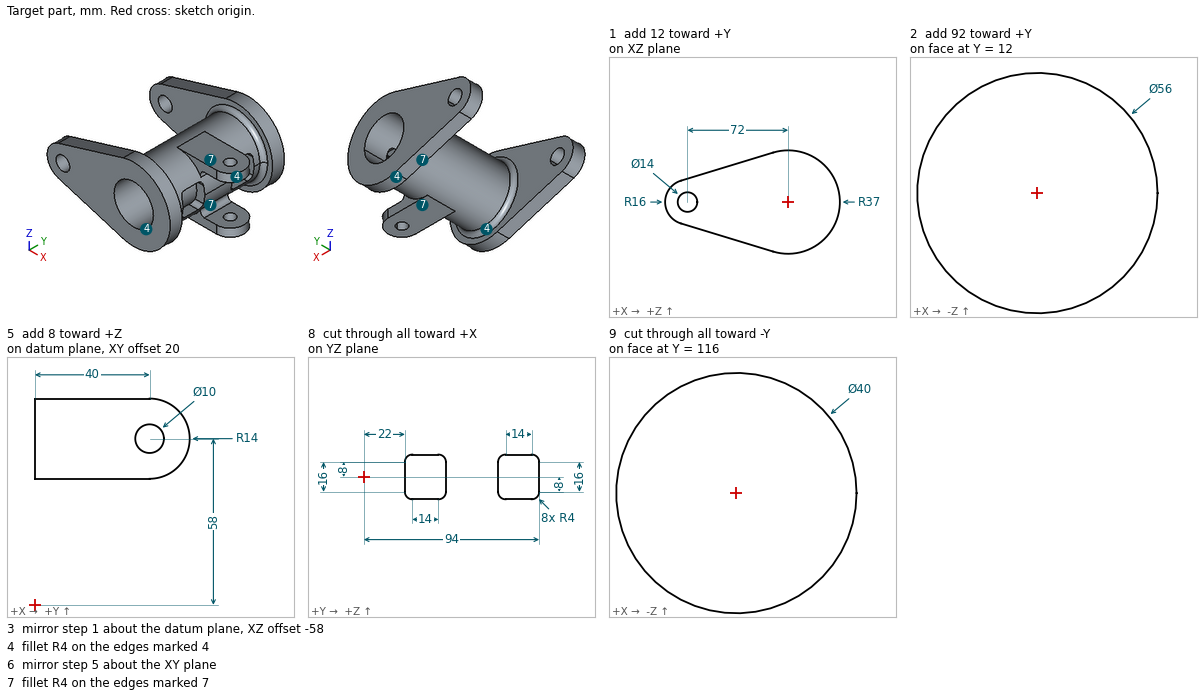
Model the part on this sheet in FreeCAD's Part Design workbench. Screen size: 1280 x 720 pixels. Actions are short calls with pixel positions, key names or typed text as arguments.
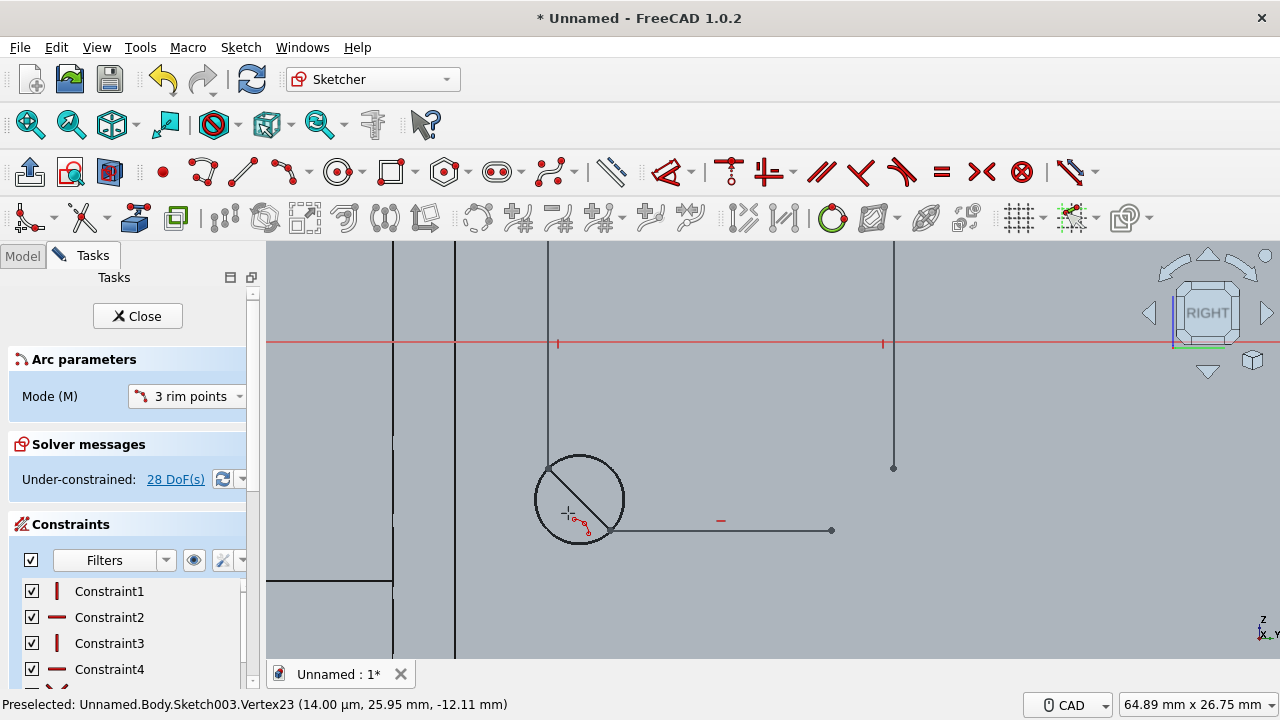
click(568, 511)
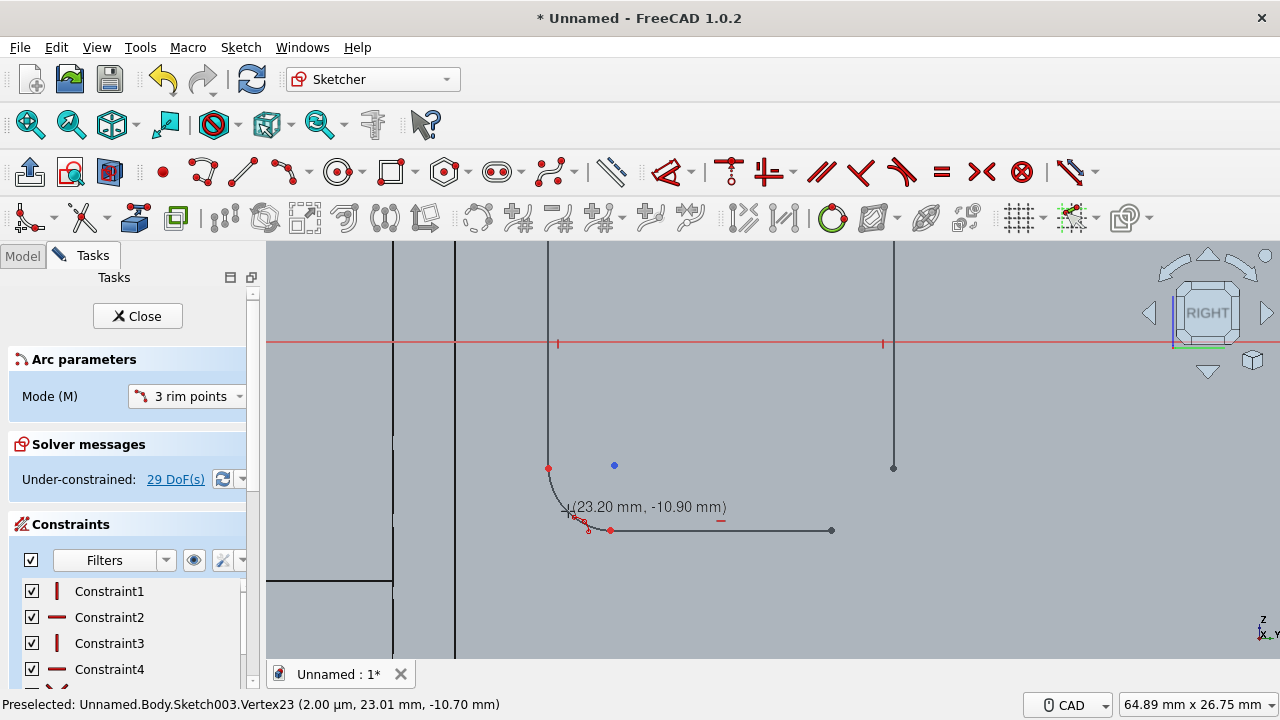
click(831, 531)
click(894, 468)
click(875, 511)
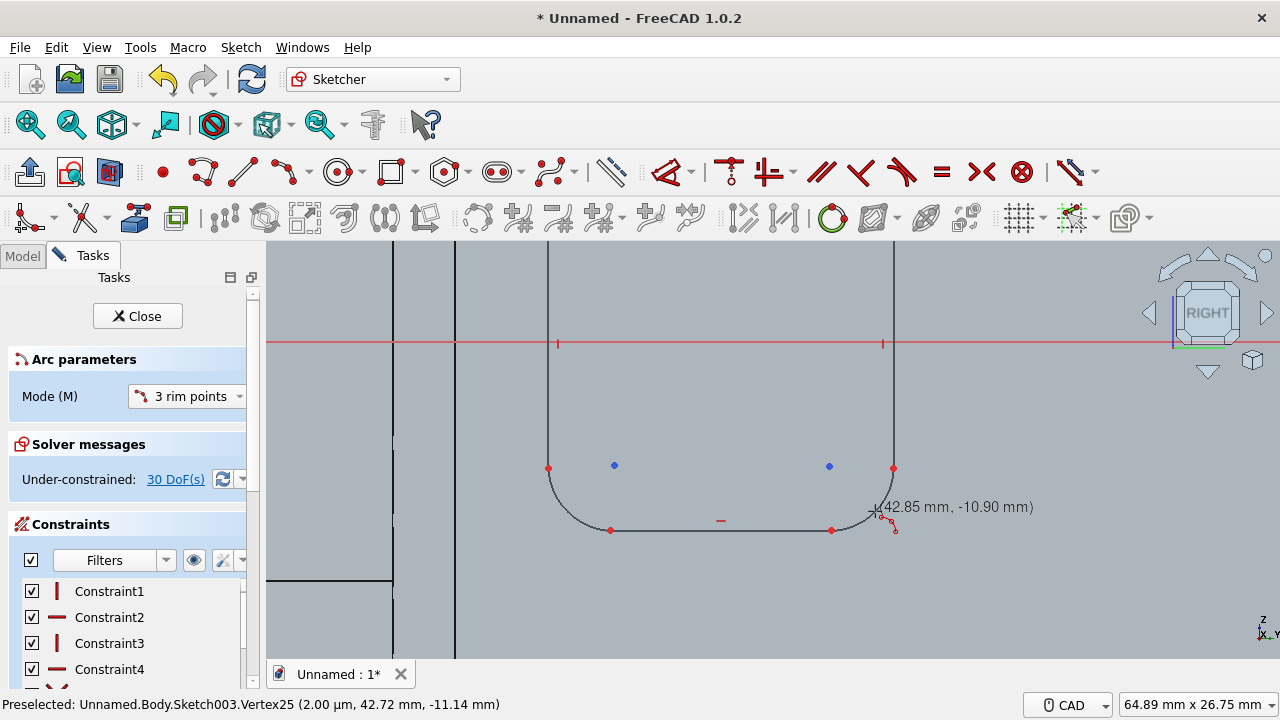
scroll(567, 513, down, 5)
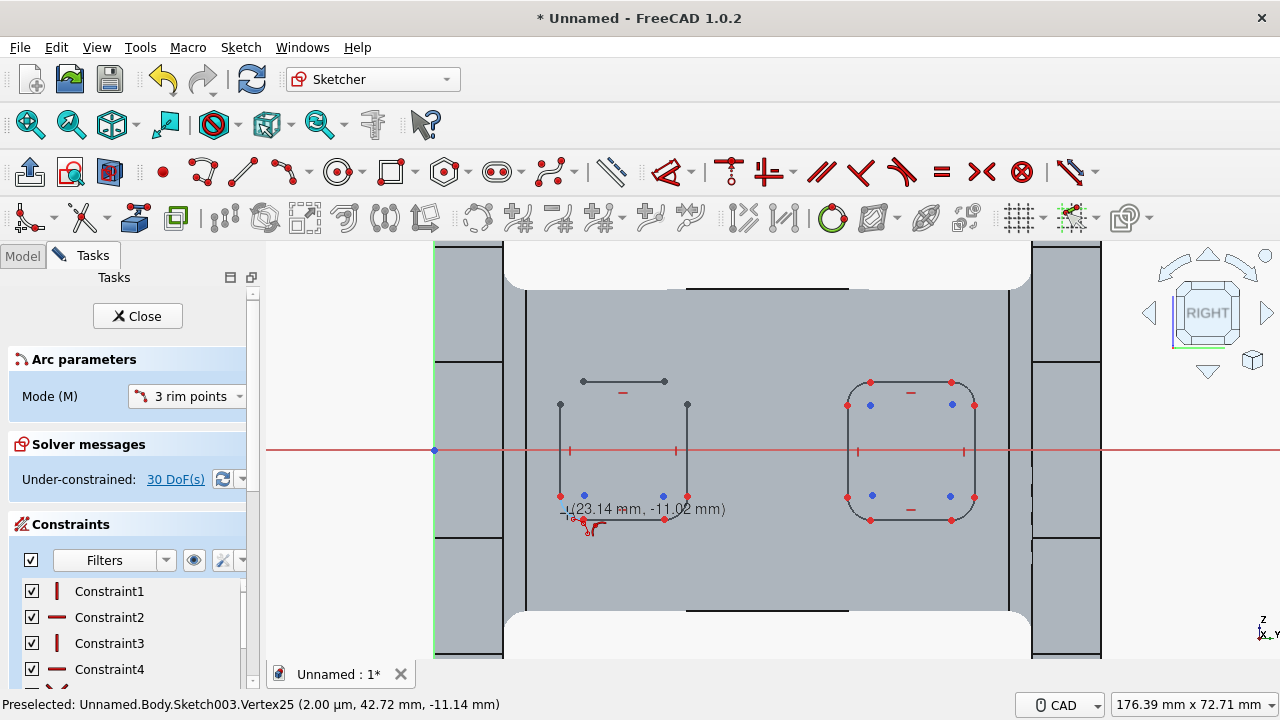
click(687, 405)
click(664, 382)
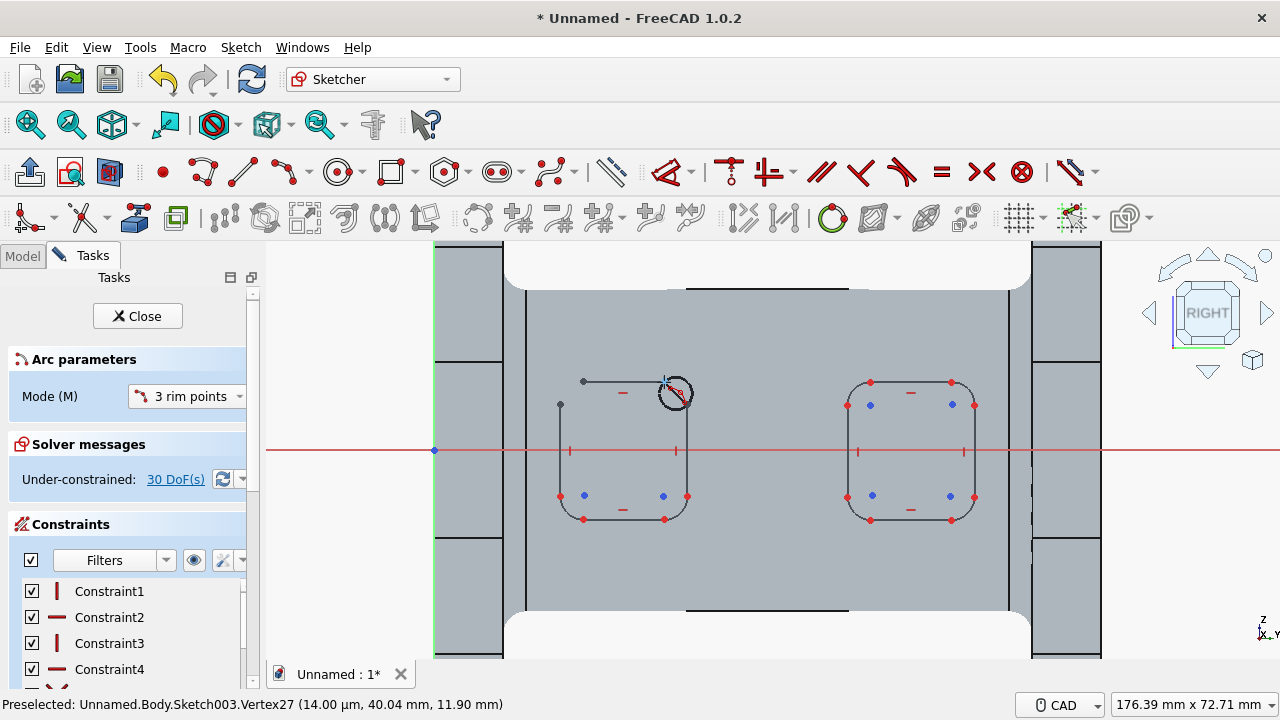
scroll(680, 388, up, 5)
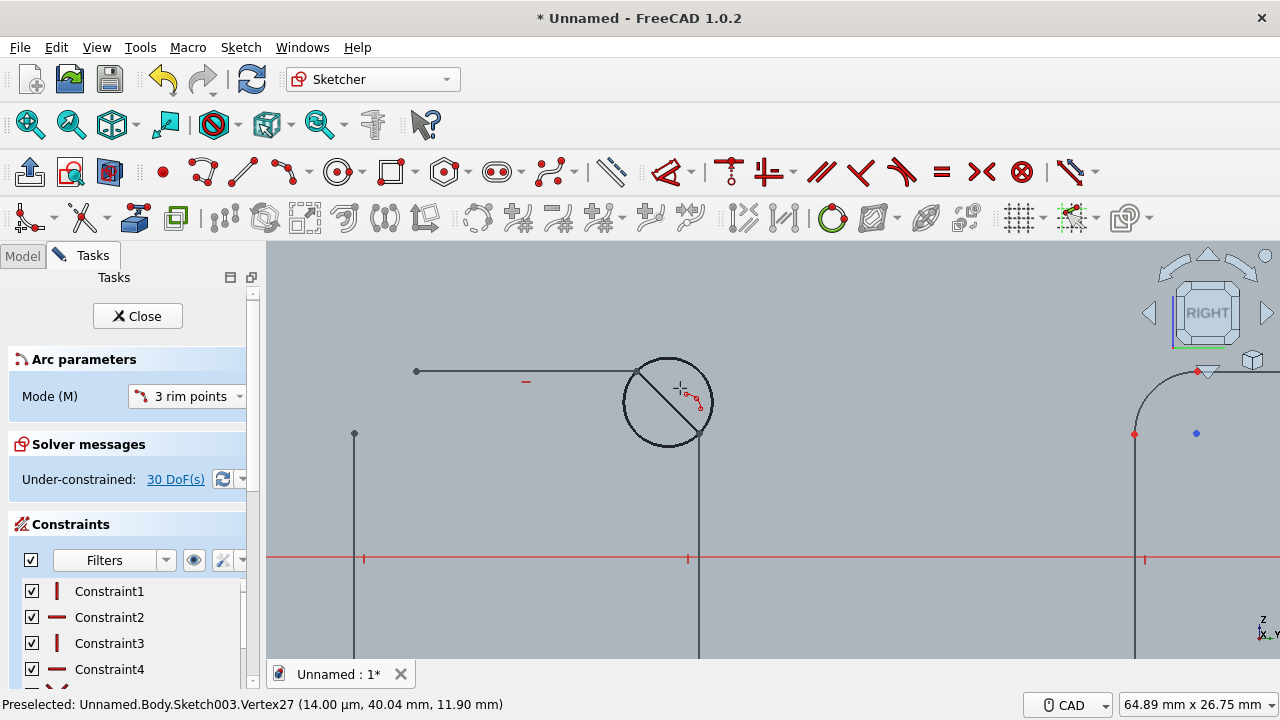
click(680, 388)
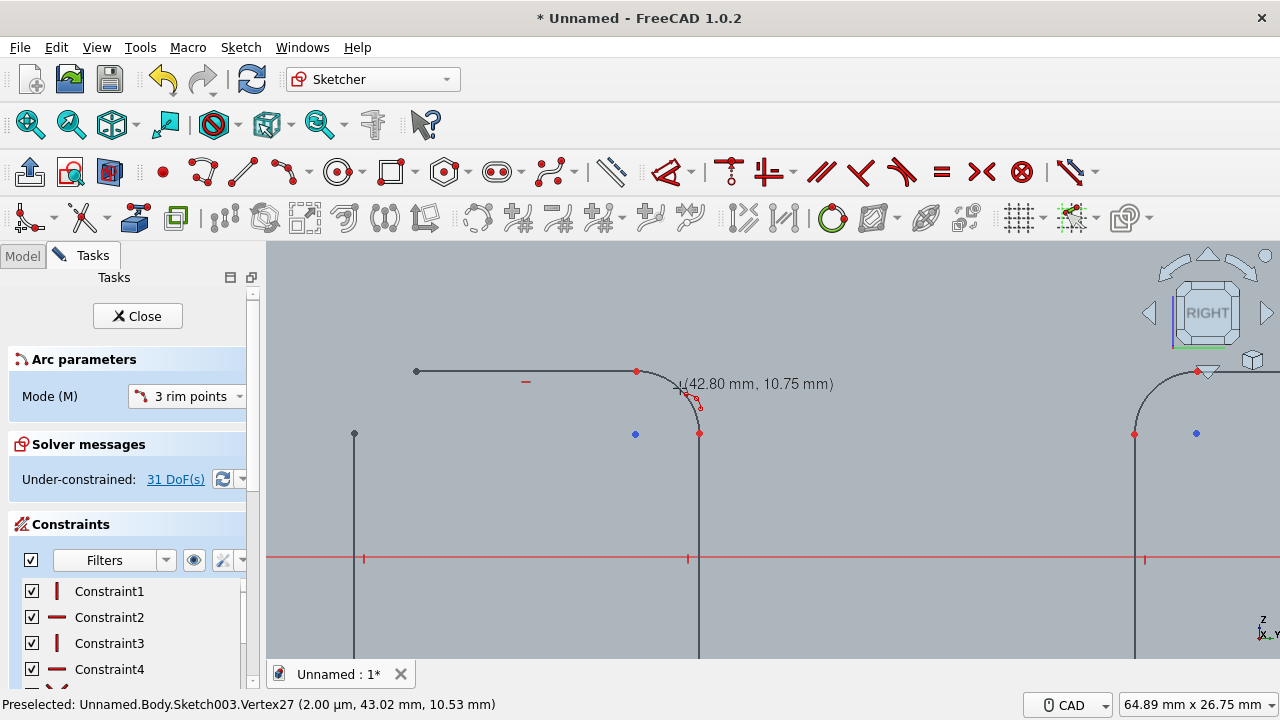
click(417, 371)
click(354, 434)
click(373, 388)
key(Escape)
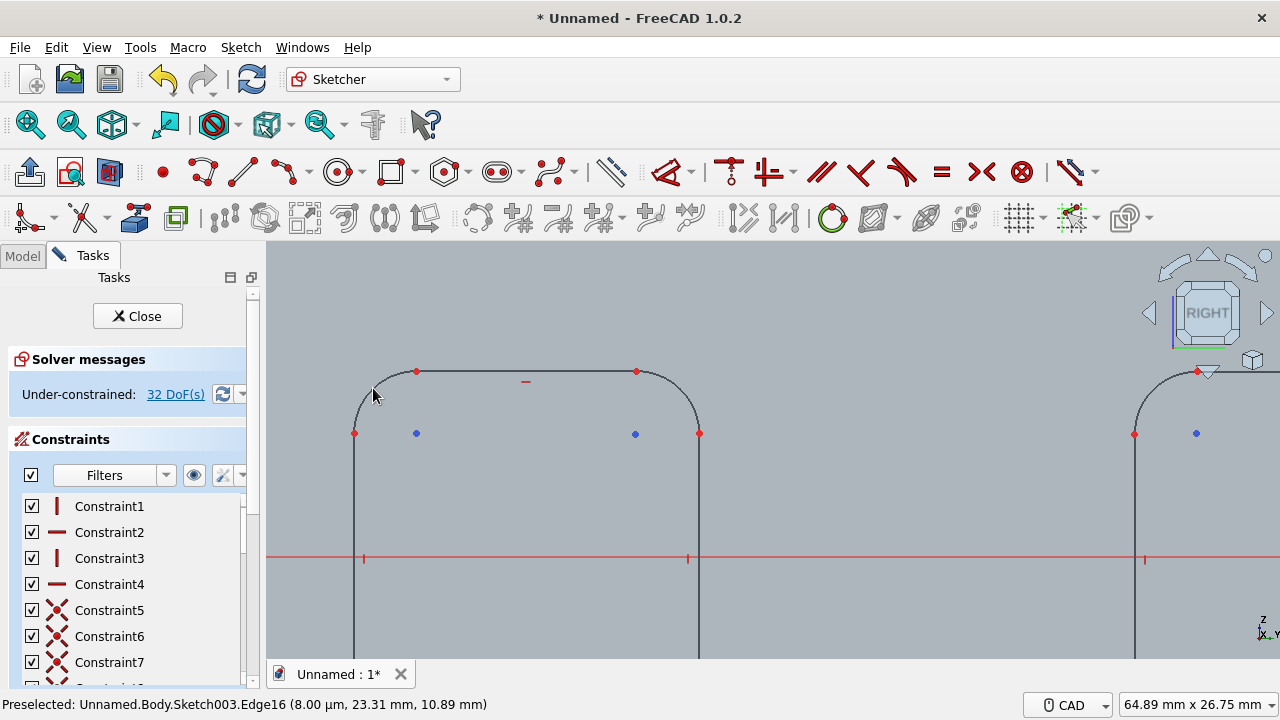
scroll(681, 388, down, 5)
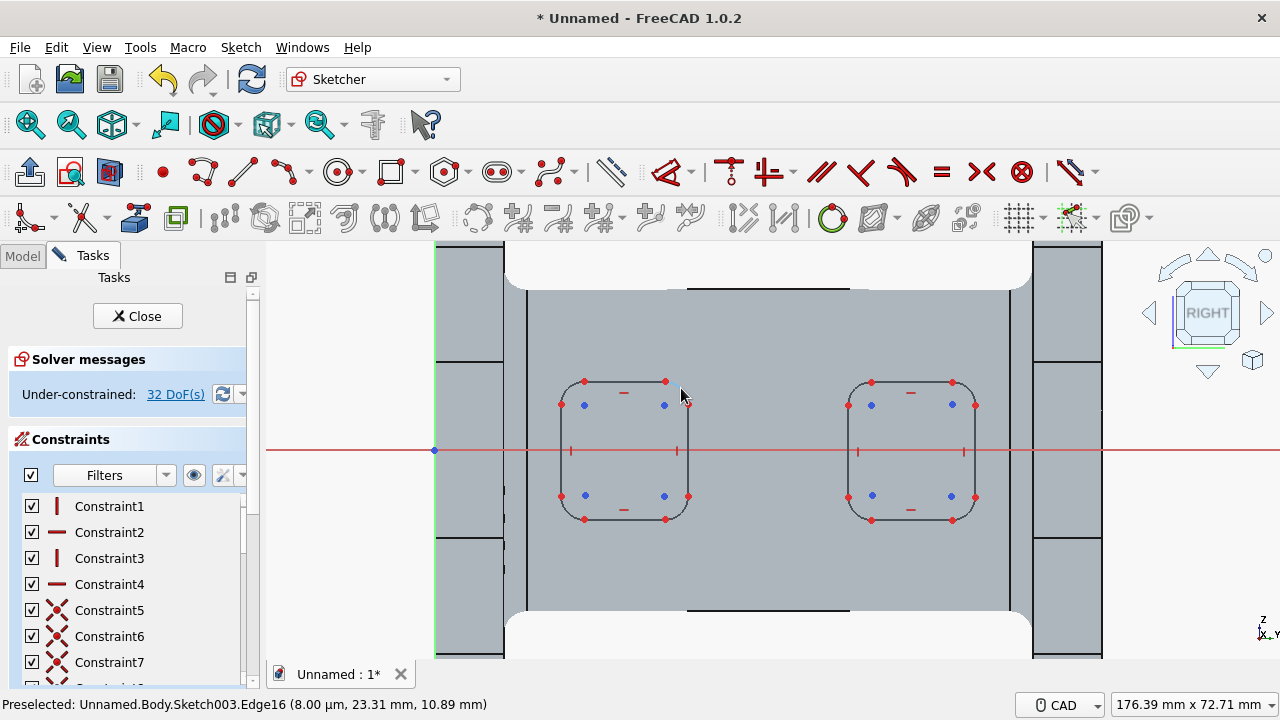
click(975, 470)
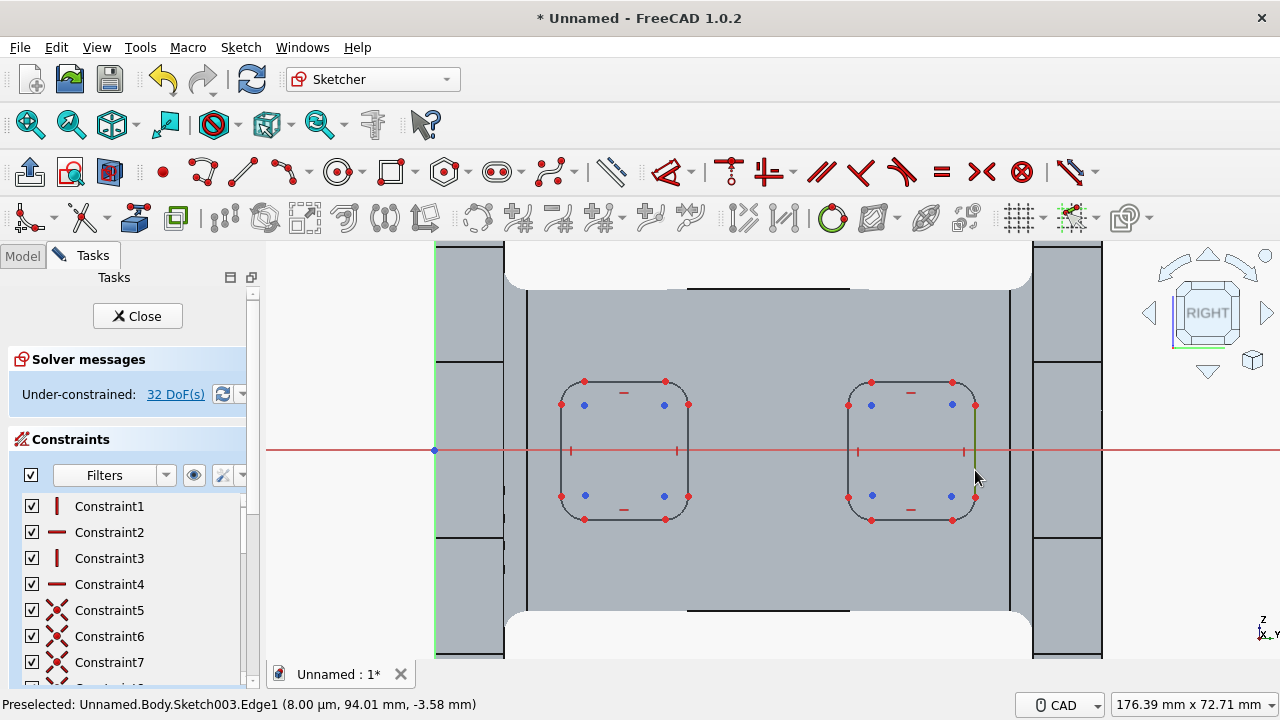
scroll(973, 395, up, 2)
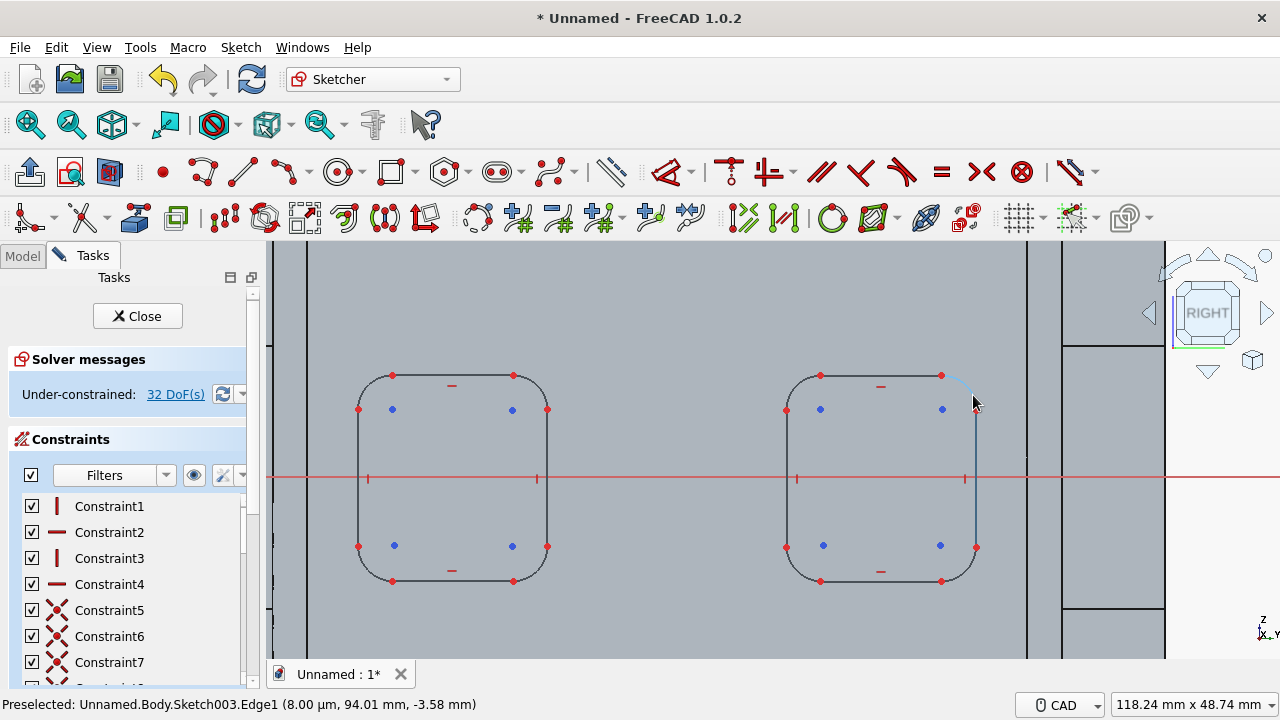
click(973, 394)